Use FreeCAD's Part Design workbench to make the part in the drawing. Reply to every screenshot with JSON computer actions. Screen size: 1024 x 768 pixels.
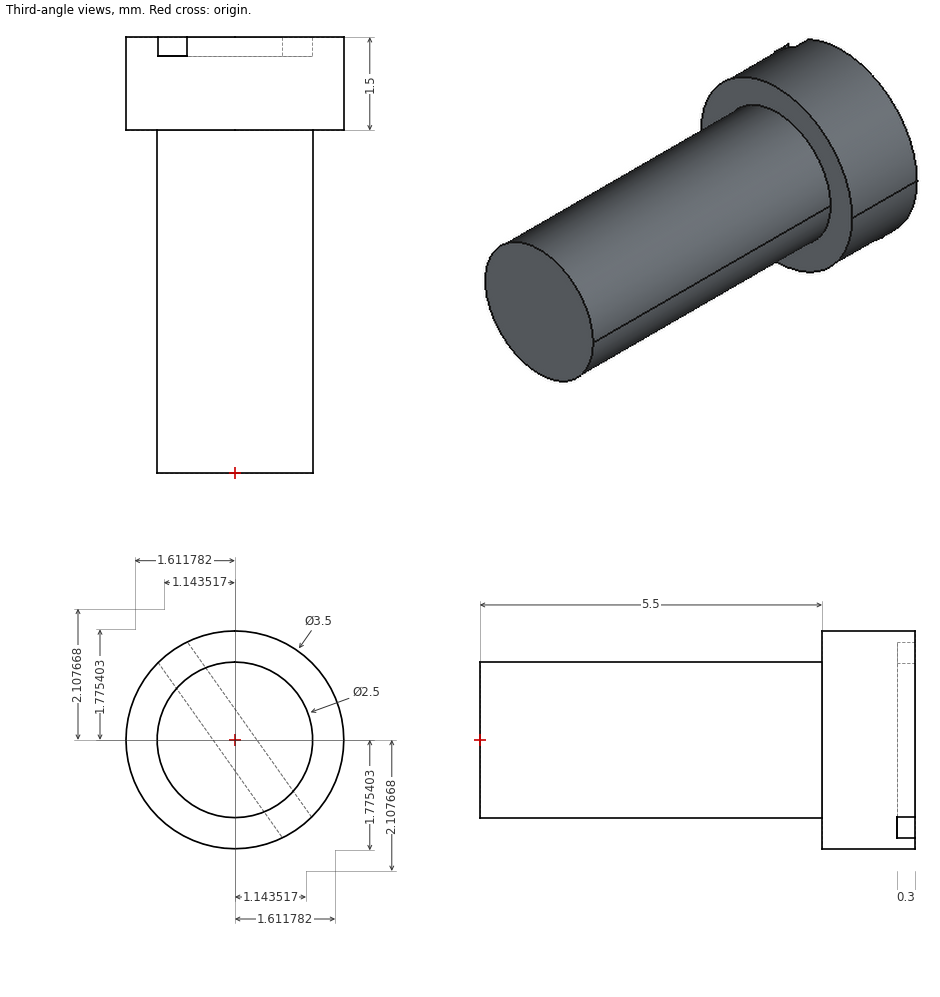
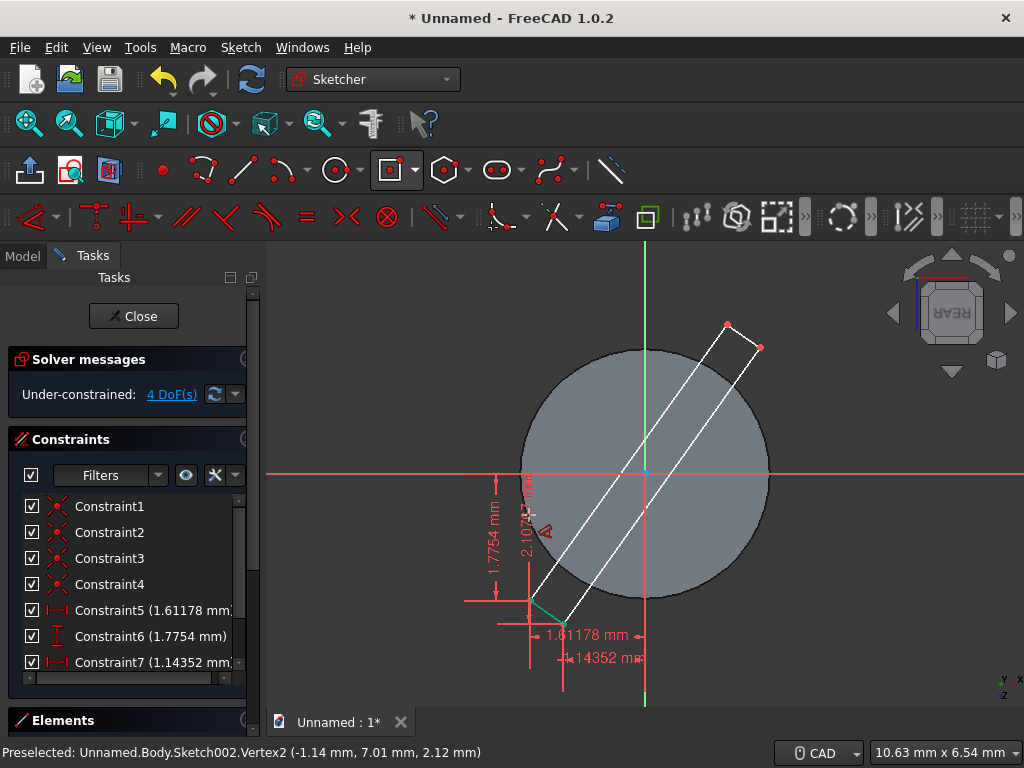
{"action": "left_click", "coordinate": [760, 348]}
{"action": "left_click", "coordinate": [702, 314]}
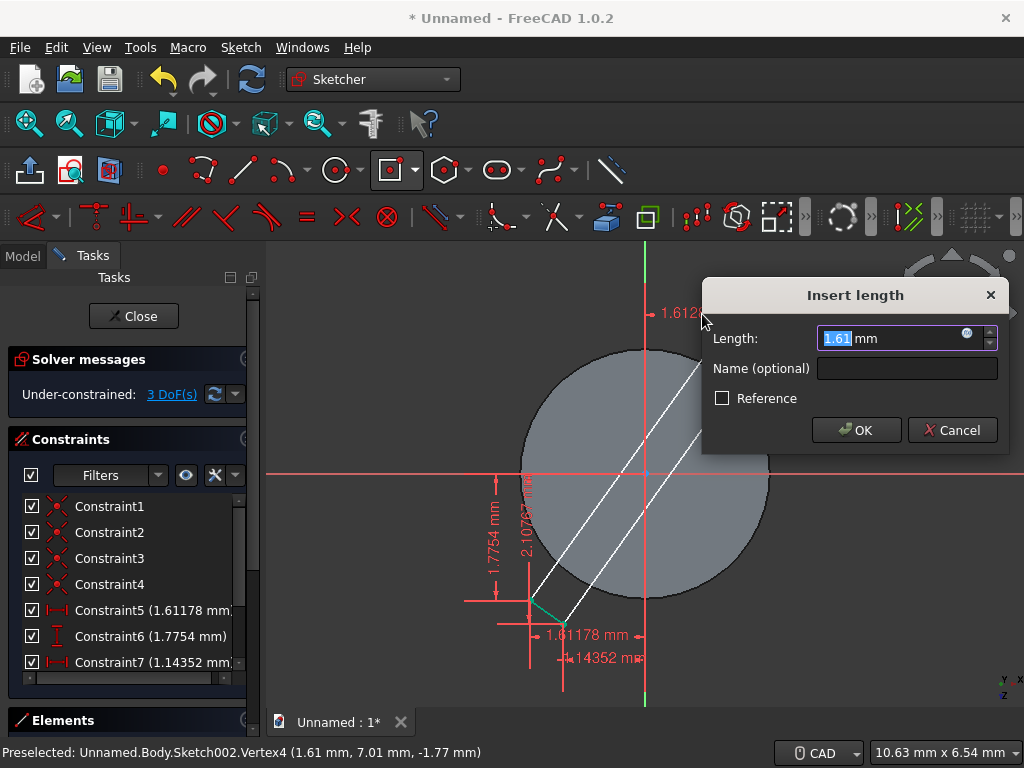
{"action": "type", "text": "1.611782"}
{"action": "key", "text": "Return"}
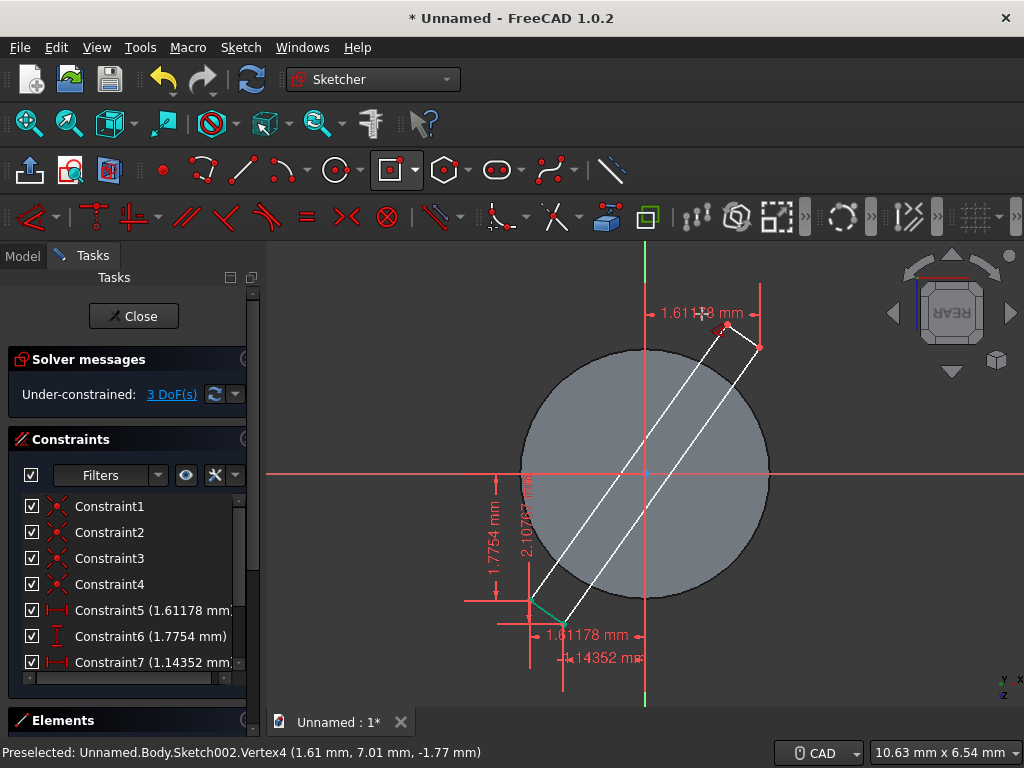
{"action": "left_click", "coordinate": [760, 348]}
{"action": "left_click", "coordinate": [794, 411]}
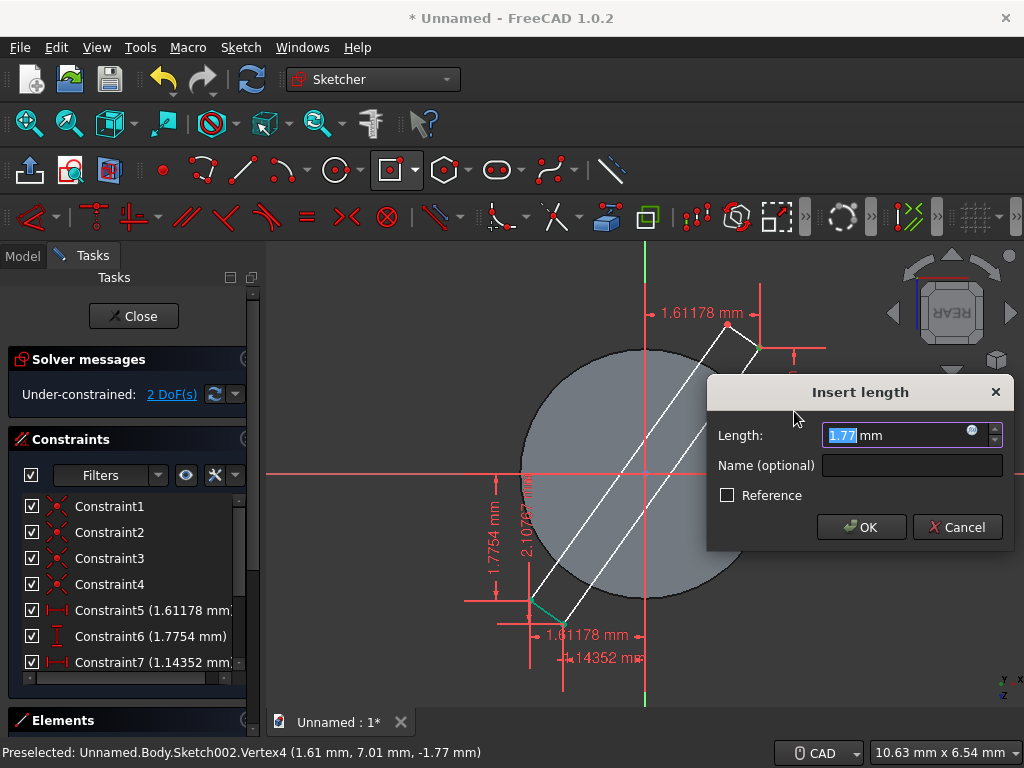
{"action": "type", "text": "1.775403"}
{"action": "key", "text": "Return"}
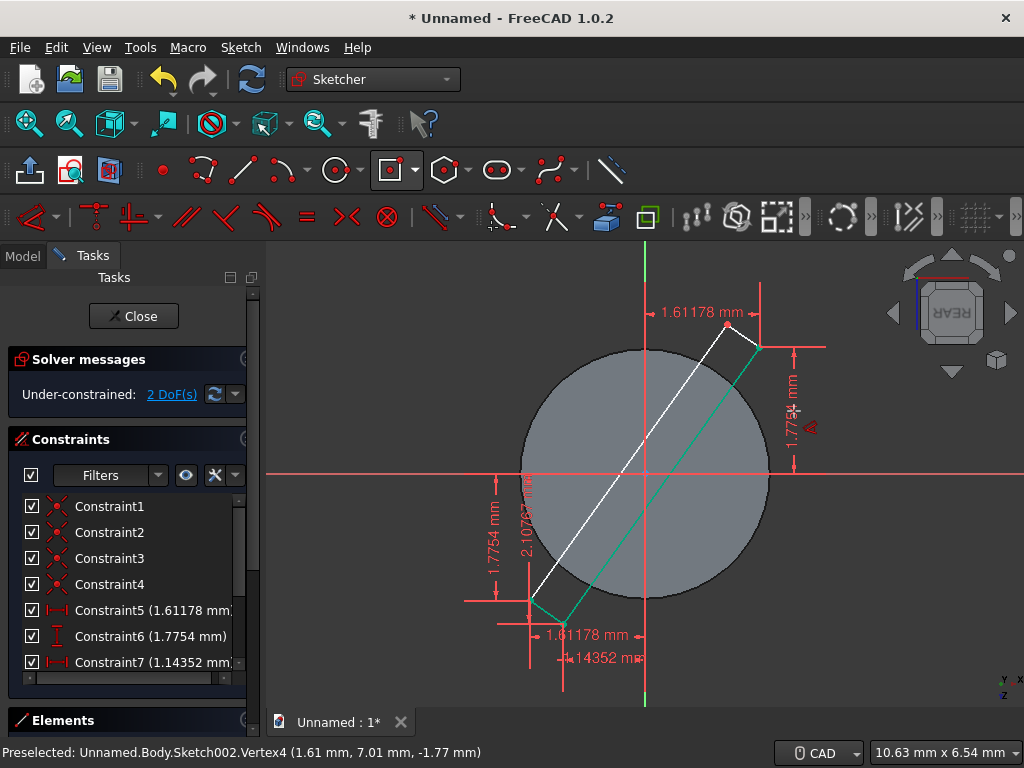
{"action": "left_click", "coordinate": [727, 325]}
{"action": "left_click", "coordinate": [686, 291]}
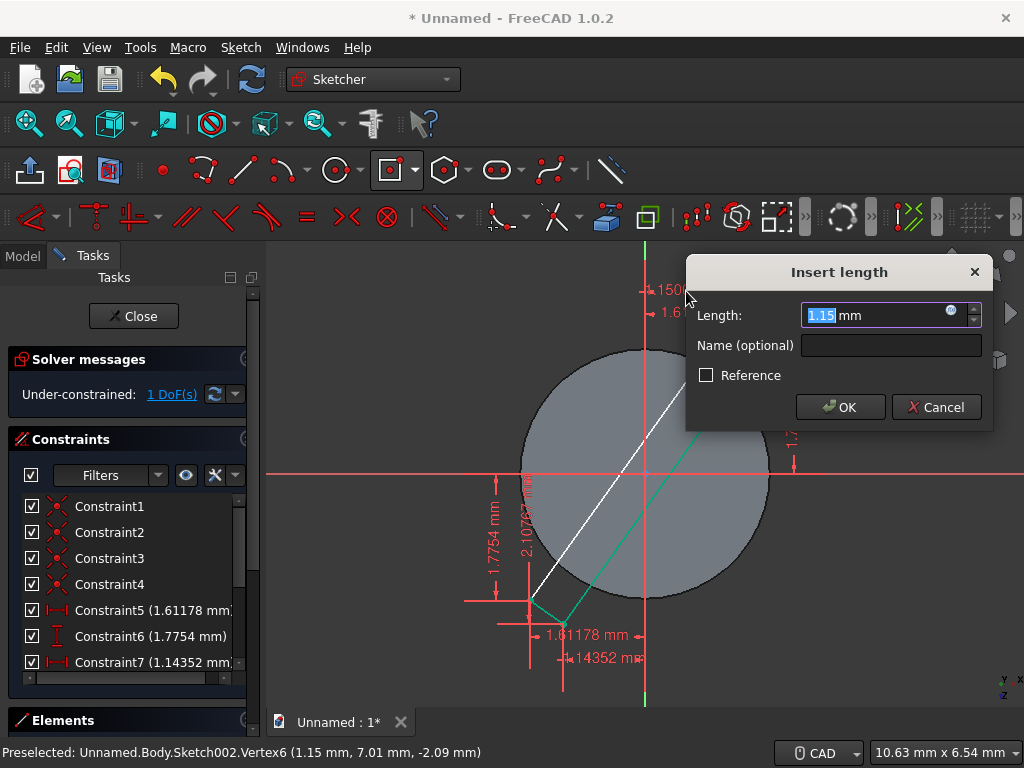
{"action": "type", "text": "1.143517"}
{"action": "key", "text": "Return"}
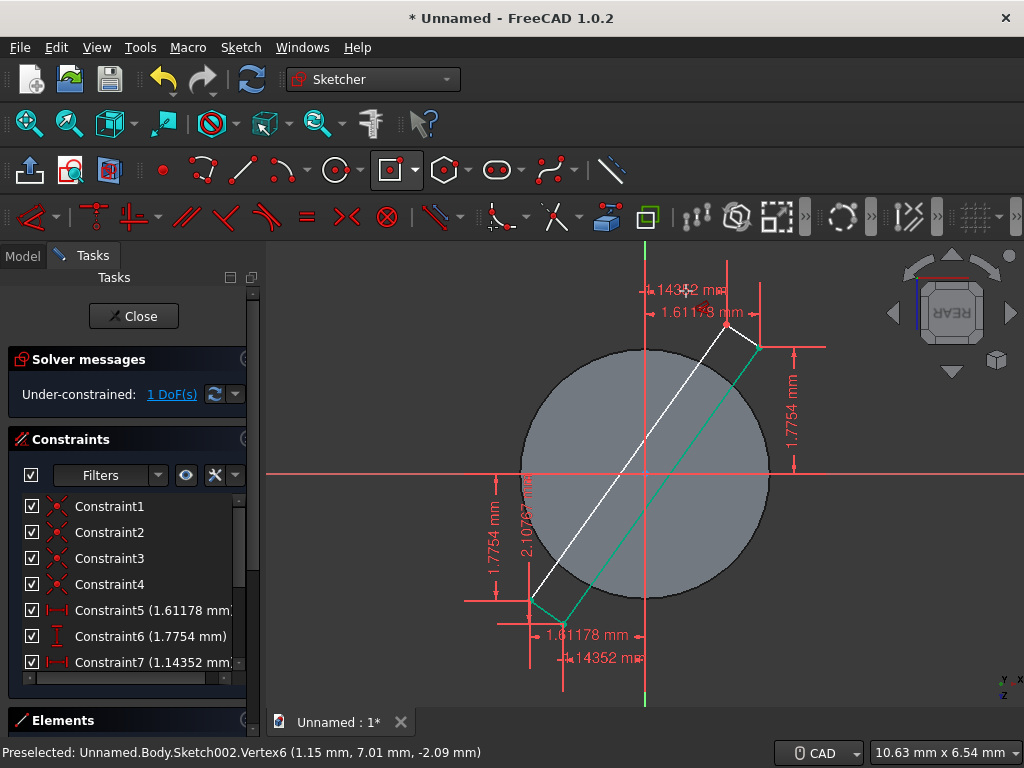
{"action": "left_click", "coordinate": [727, 325]}
{"action": "left_click", "coordinate": [761, 434]}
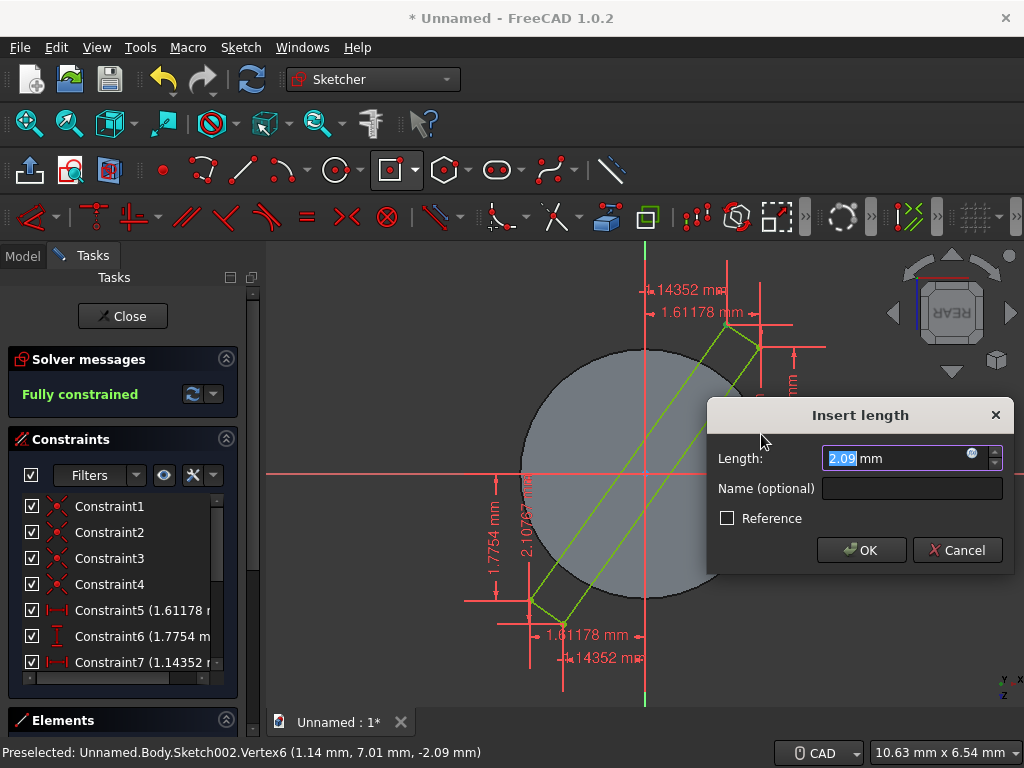
{"action": "type", "text": "2.107668"}
{"action": "key", "text": "Return"}
{"action": "key", "text": "Escape"}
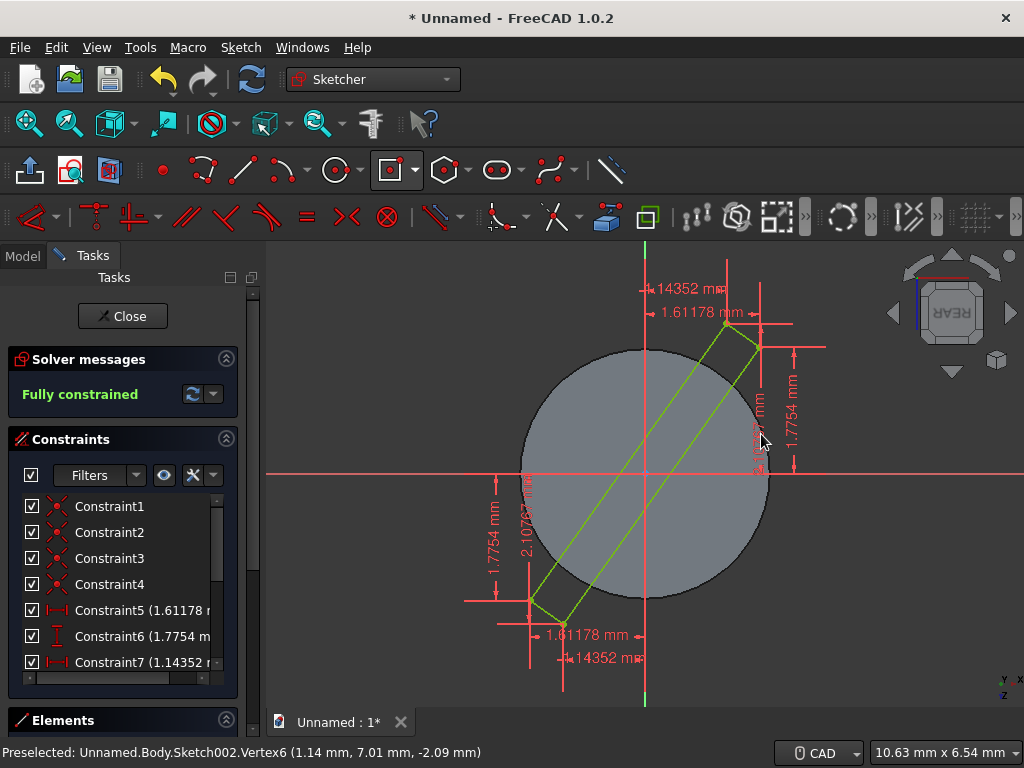
{"action": "left_click", "coordinate": [123, 316]}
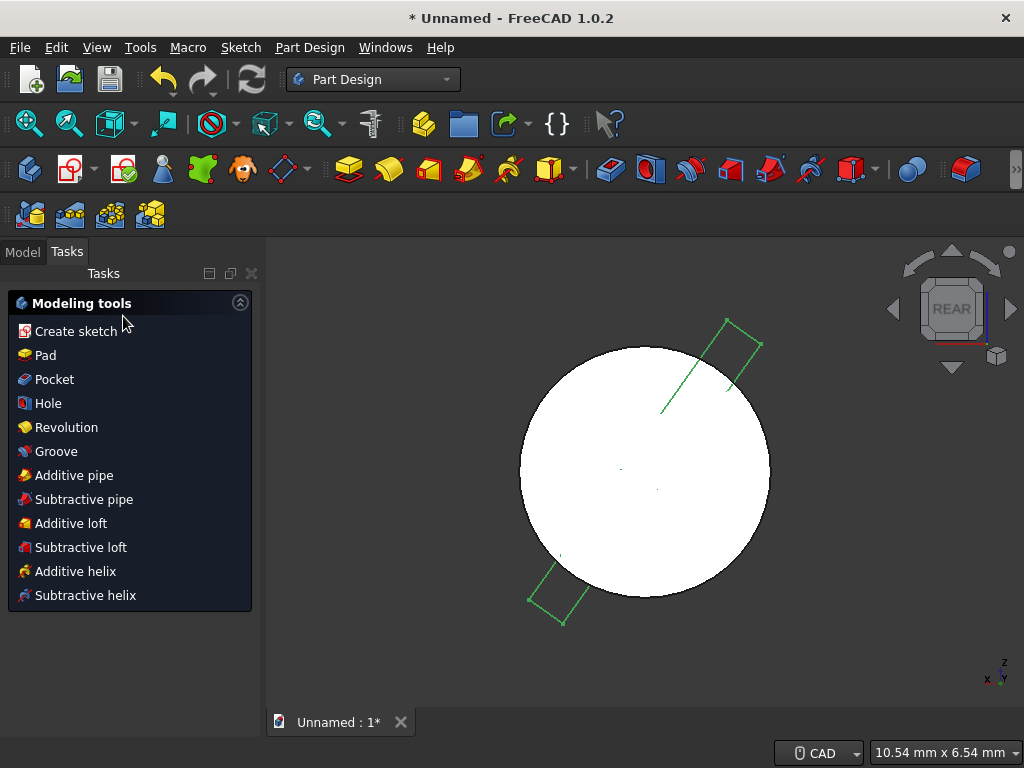
{"action": "left_click", "coordinate": [612, 170]}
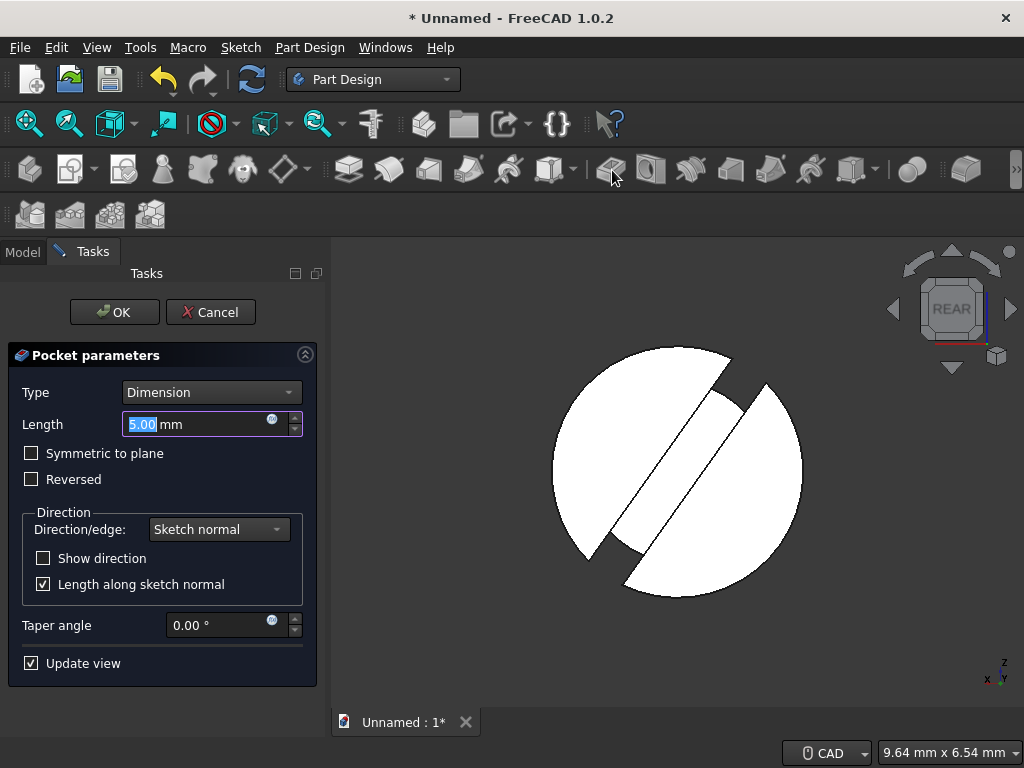
{"action": "type", "text": "0.3"}
{"action": "key", "text": "Tab"}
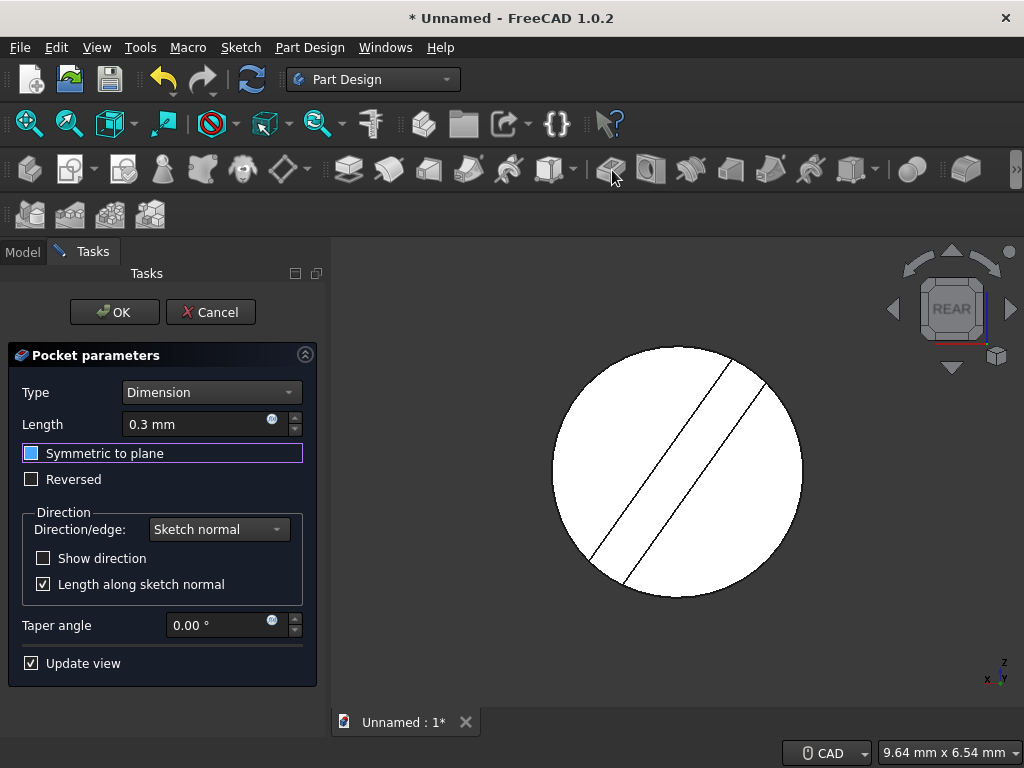
{"action": "left_click", "coordinate": [115, 312]}